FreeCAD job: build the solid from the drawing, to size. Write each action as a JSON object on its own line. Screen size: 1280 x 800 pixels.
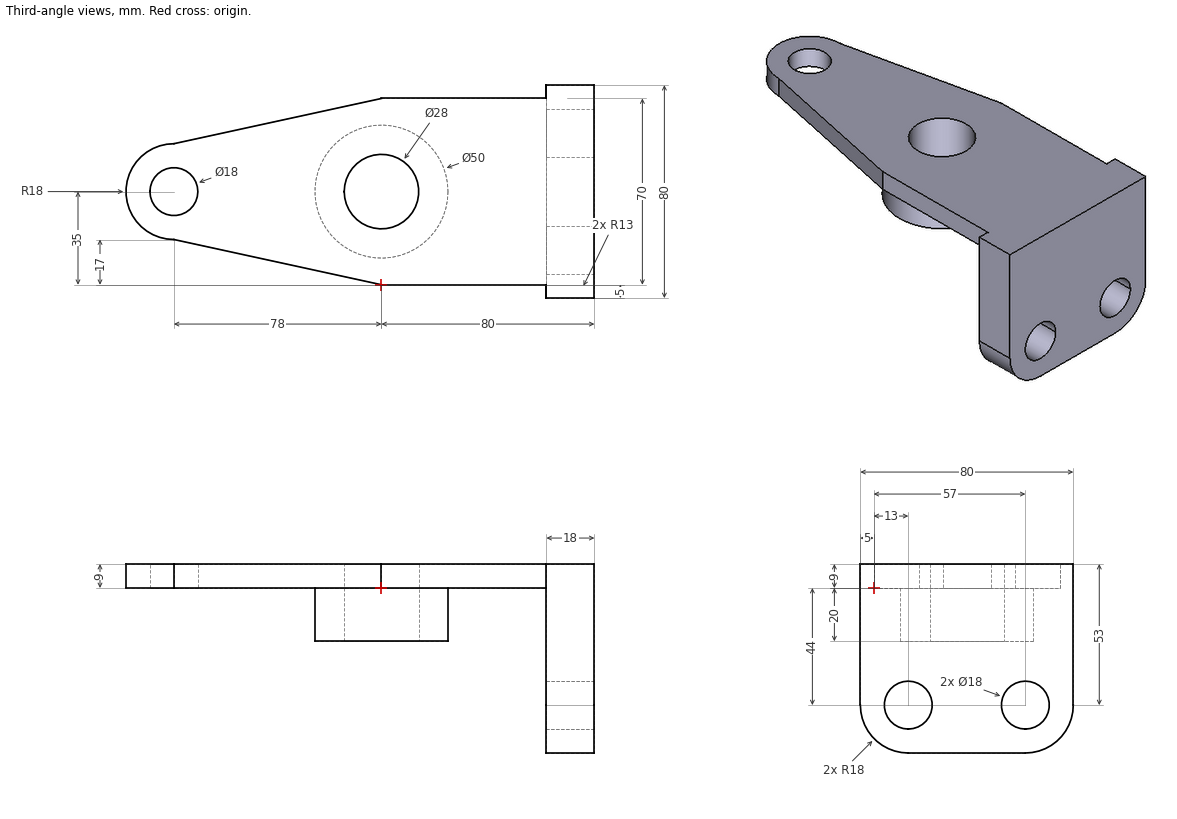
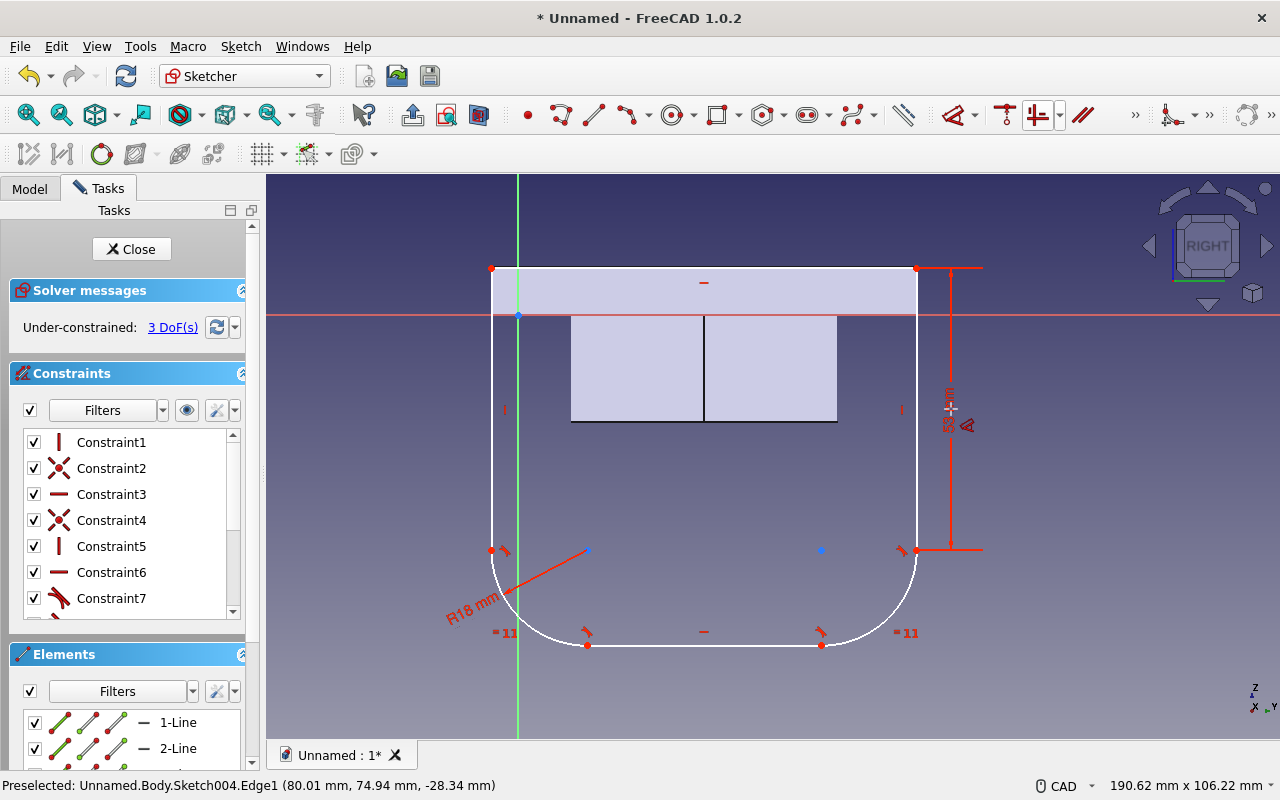
{"action": "left_click", "coordinate": [789, 268]}
{"action": "left_click", "coordinate": [704, 234]}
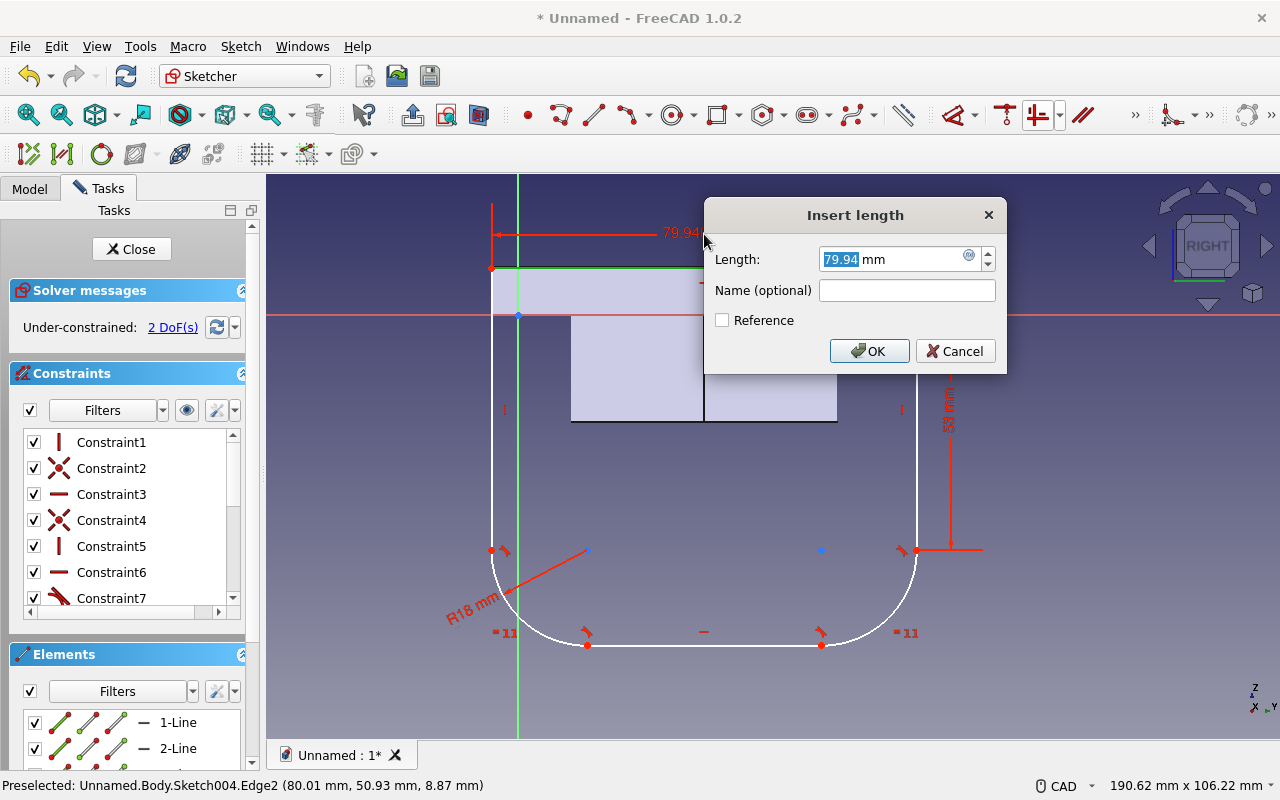
{"action": "type", "text": "80"}
{"action": "key", "text": "Return"}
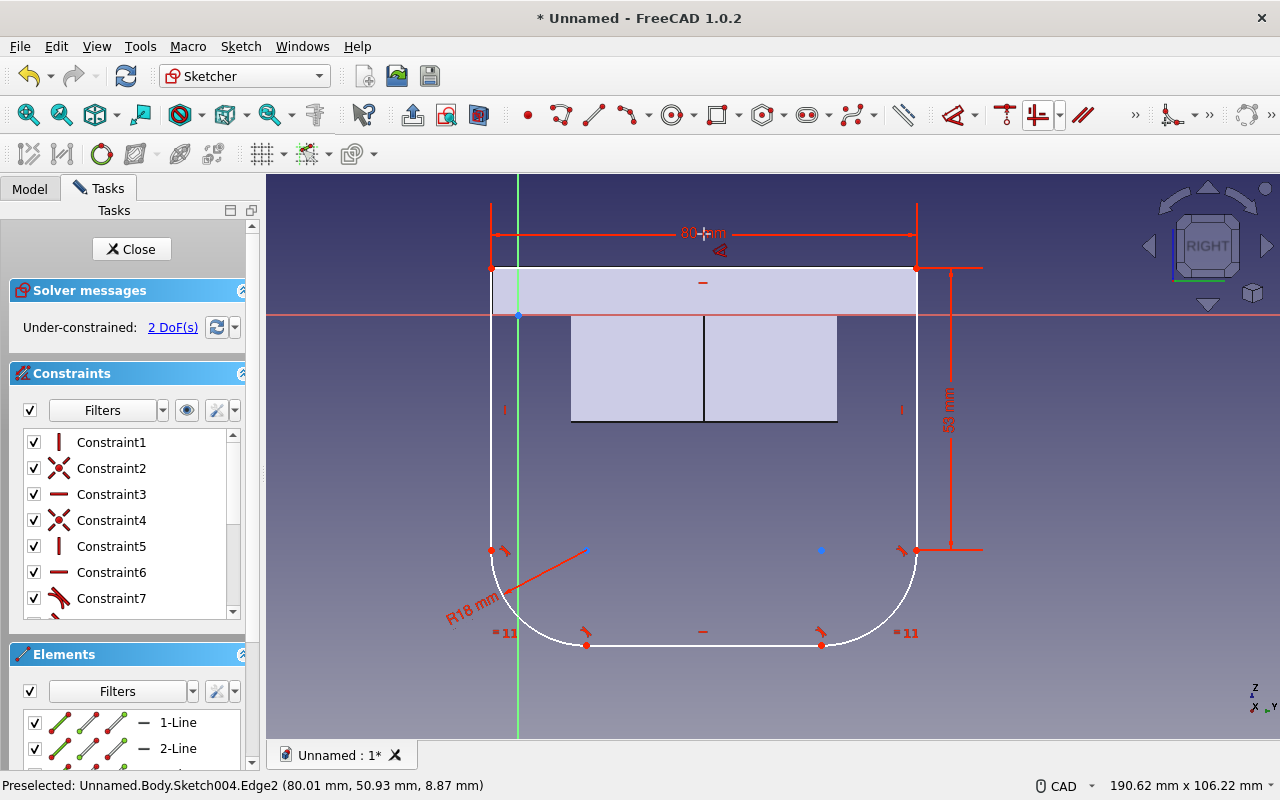
{"action": "left_click", "coordinate": [917, 268]}
{"action": "left_click", "coordinate": [951, 292]}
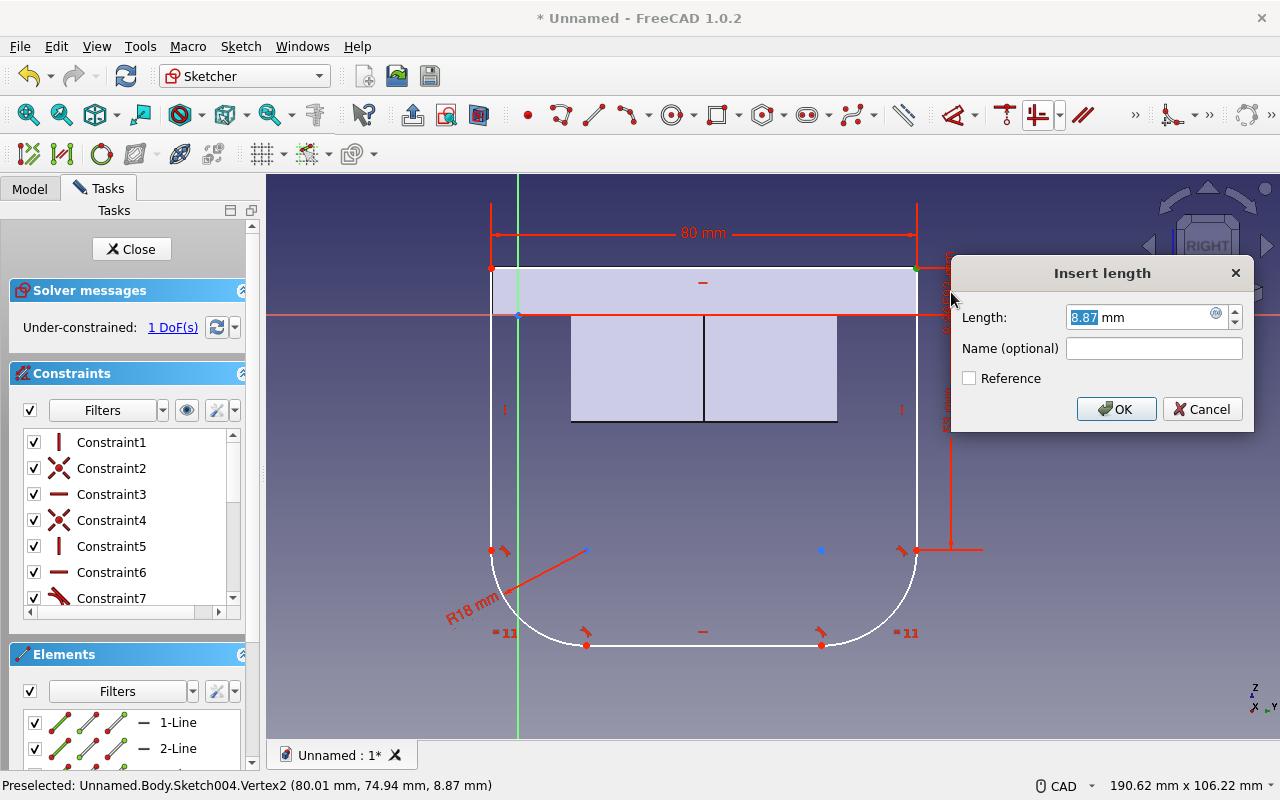
{"action": "type", "text": "9"}
{"action": "key", "text": "Return"}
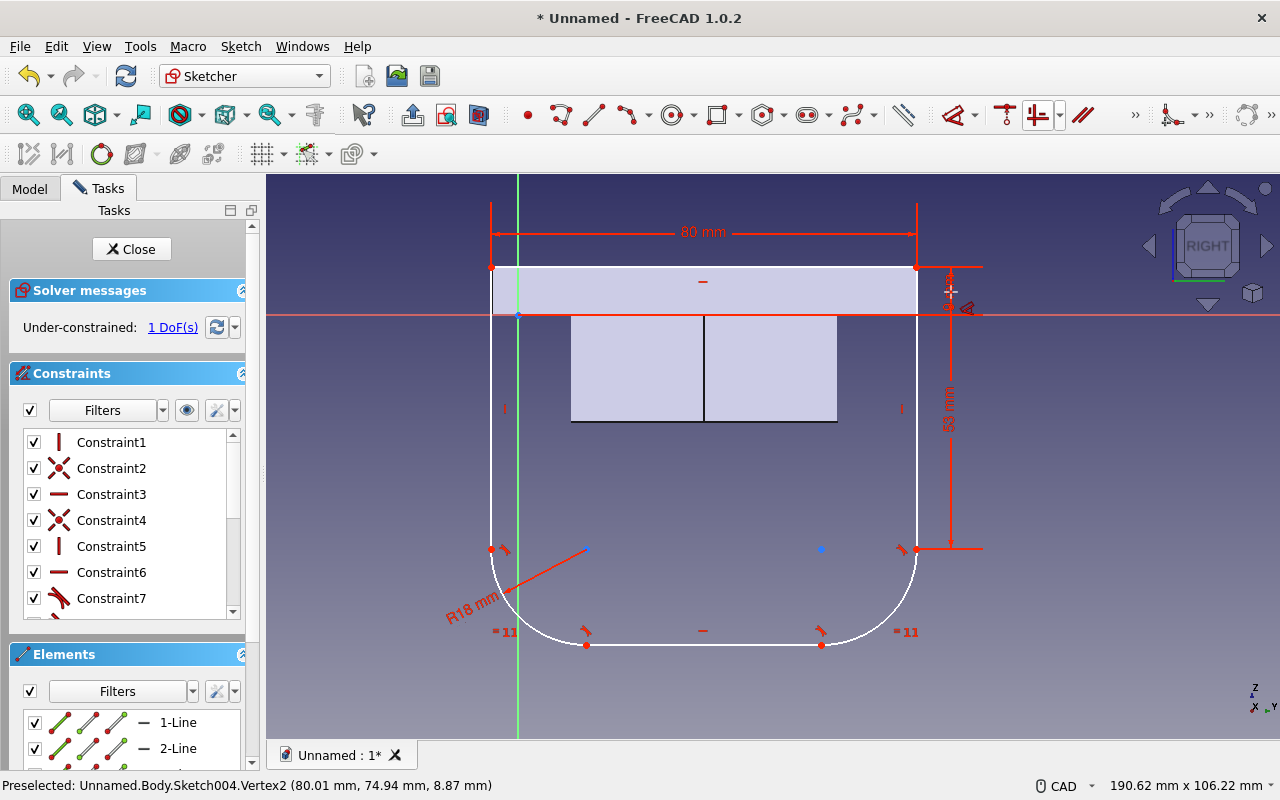
{"action": "scroll", "coordinate": [491, 267], "scroll_direction": "up", "scroll_amount": 3}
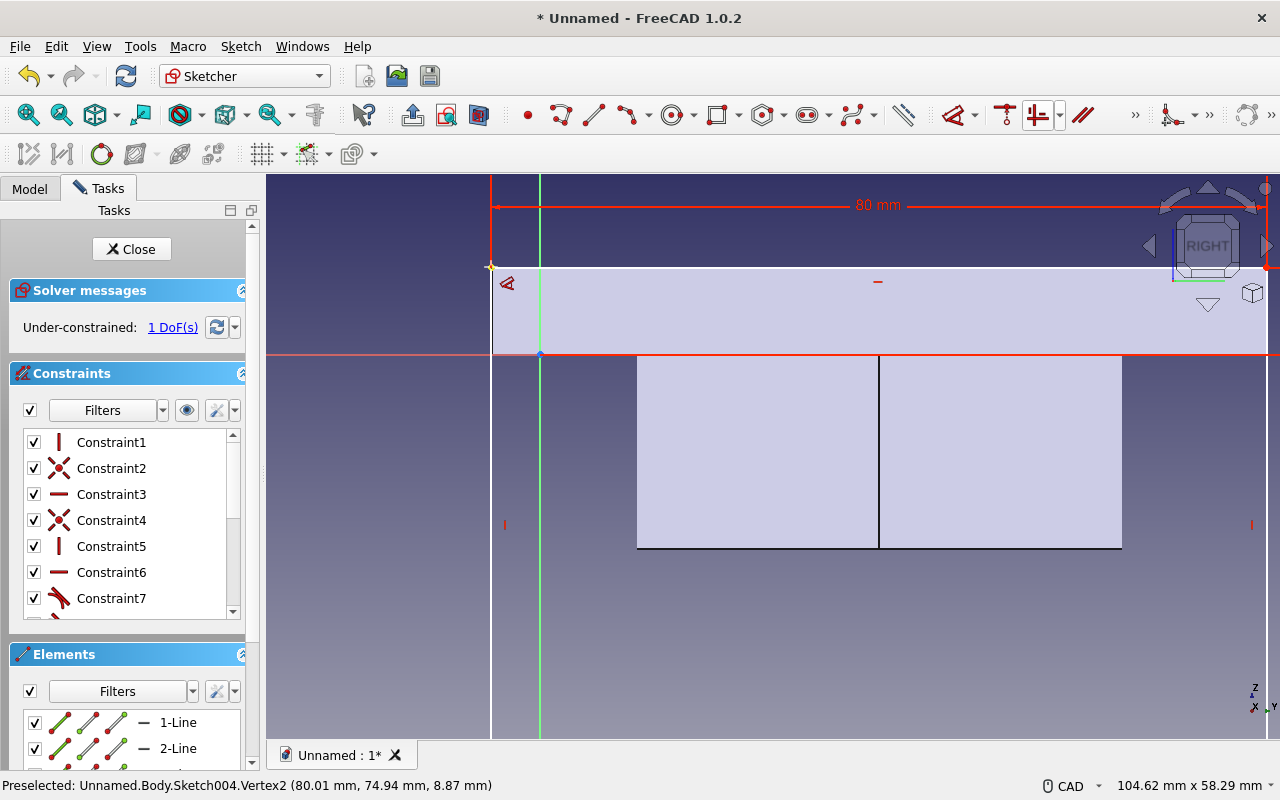
{"action": "left_click", "coordinate": [491, 268]}
{"action": "left_click", "coordinate": [516, 234]}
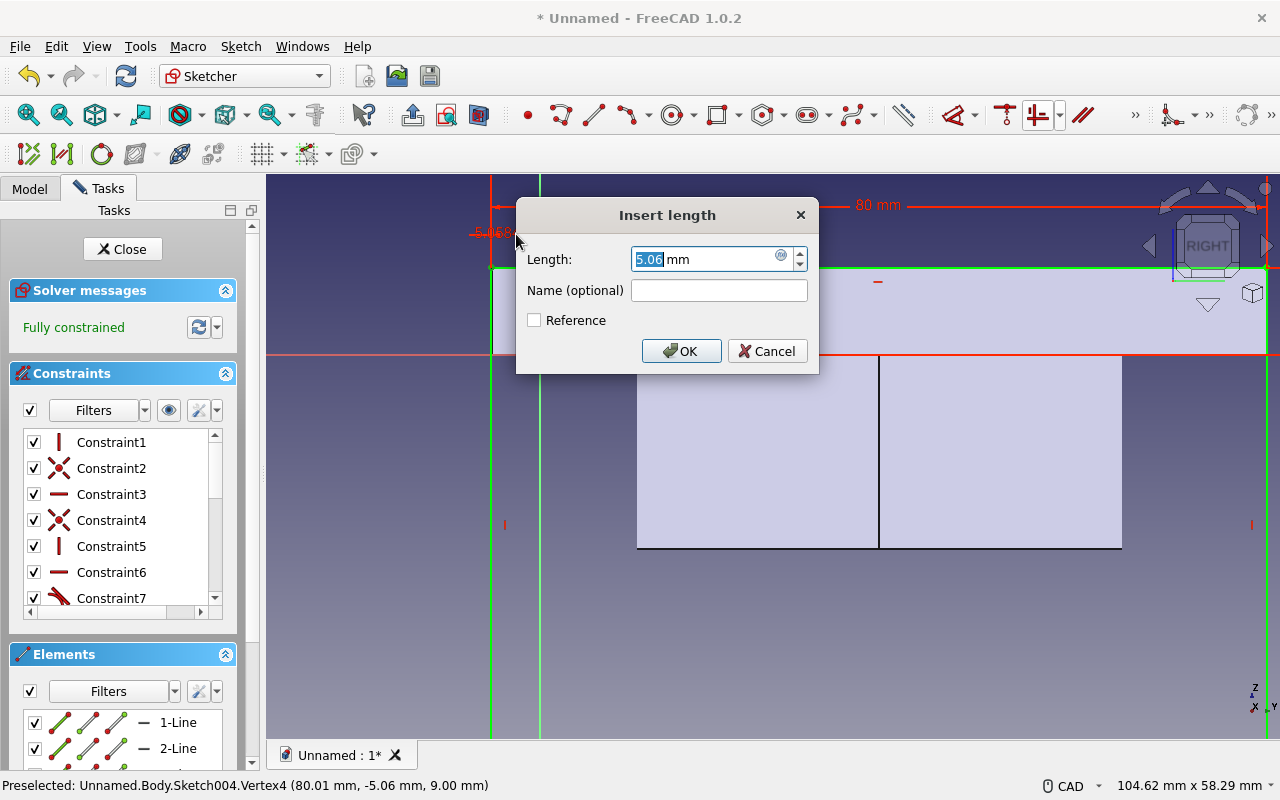
{"action": "type", "text": "5"}
{"action": "key", "text": "Return"}
{"action": "key", "text": "Escape"}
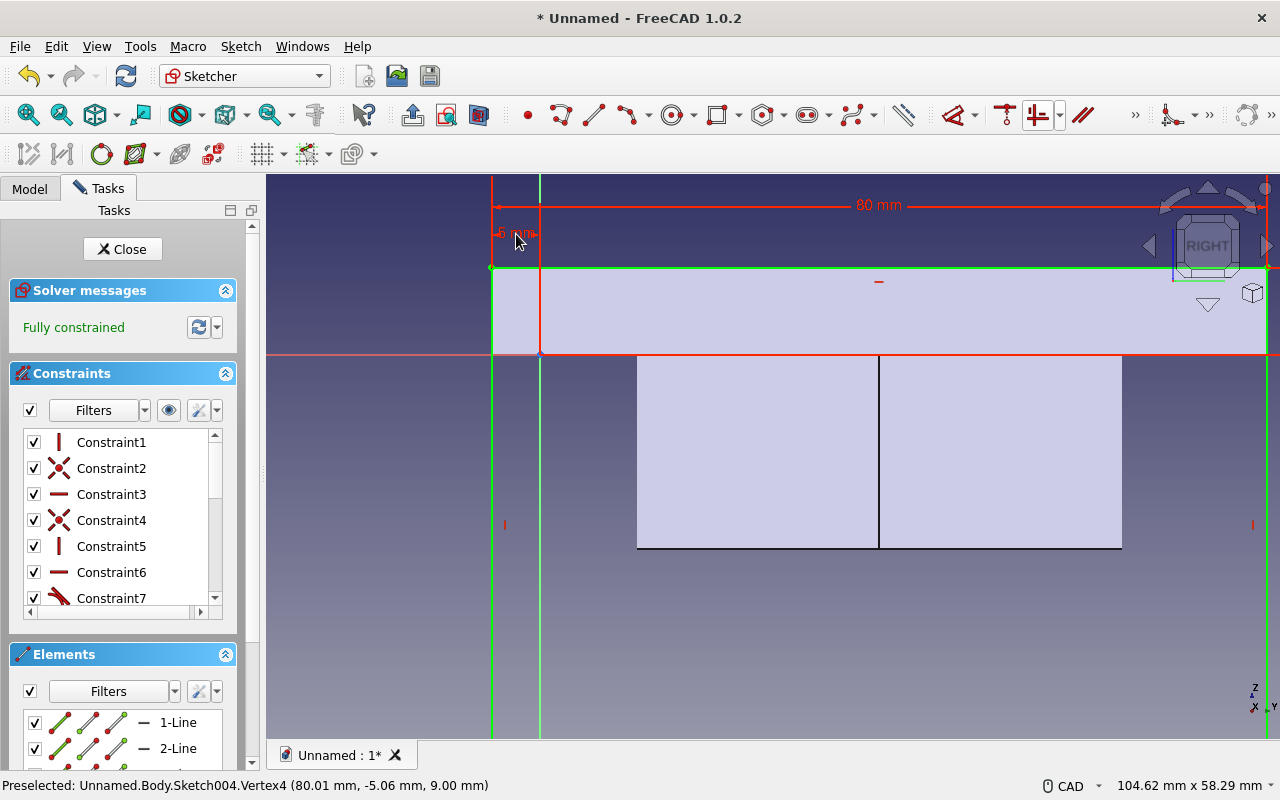
{"action": "left_click", "coordinate": [123, 249]}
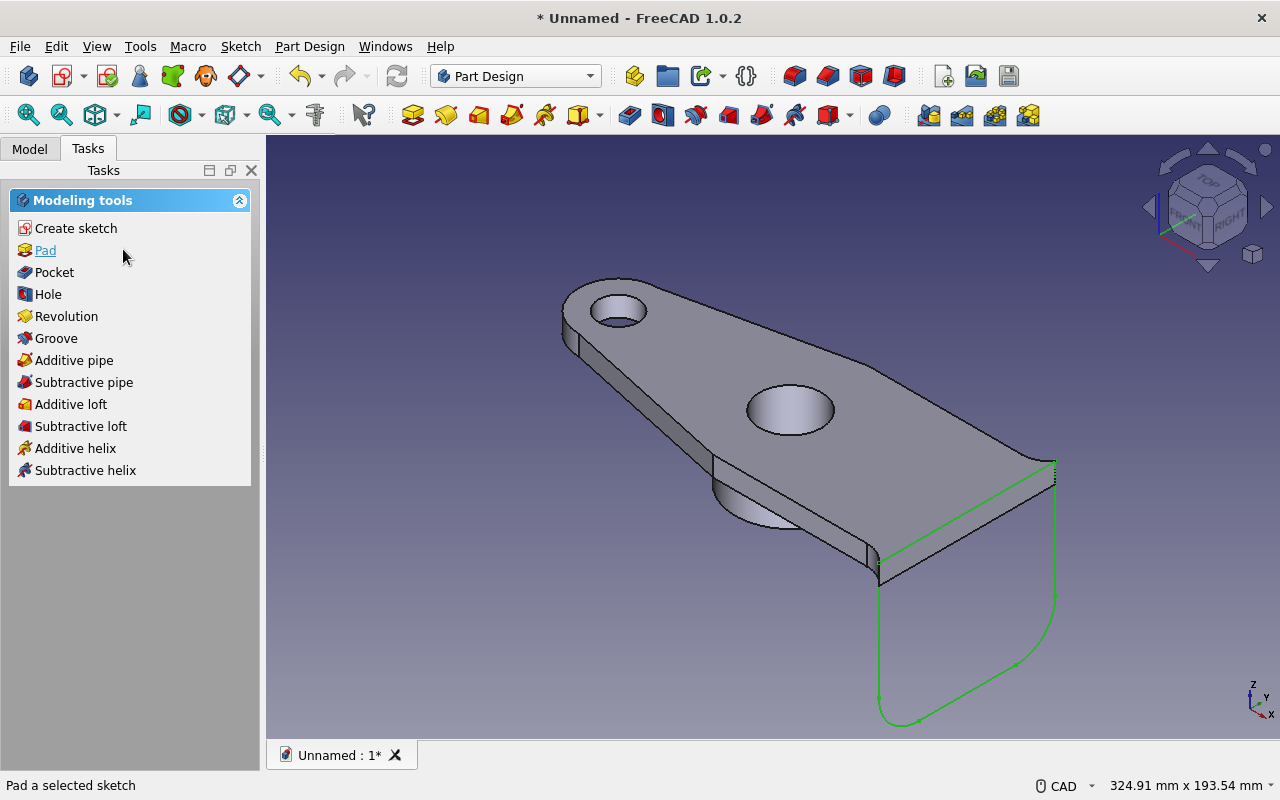
{"action": "left_click", "coordinate": [413, 116]}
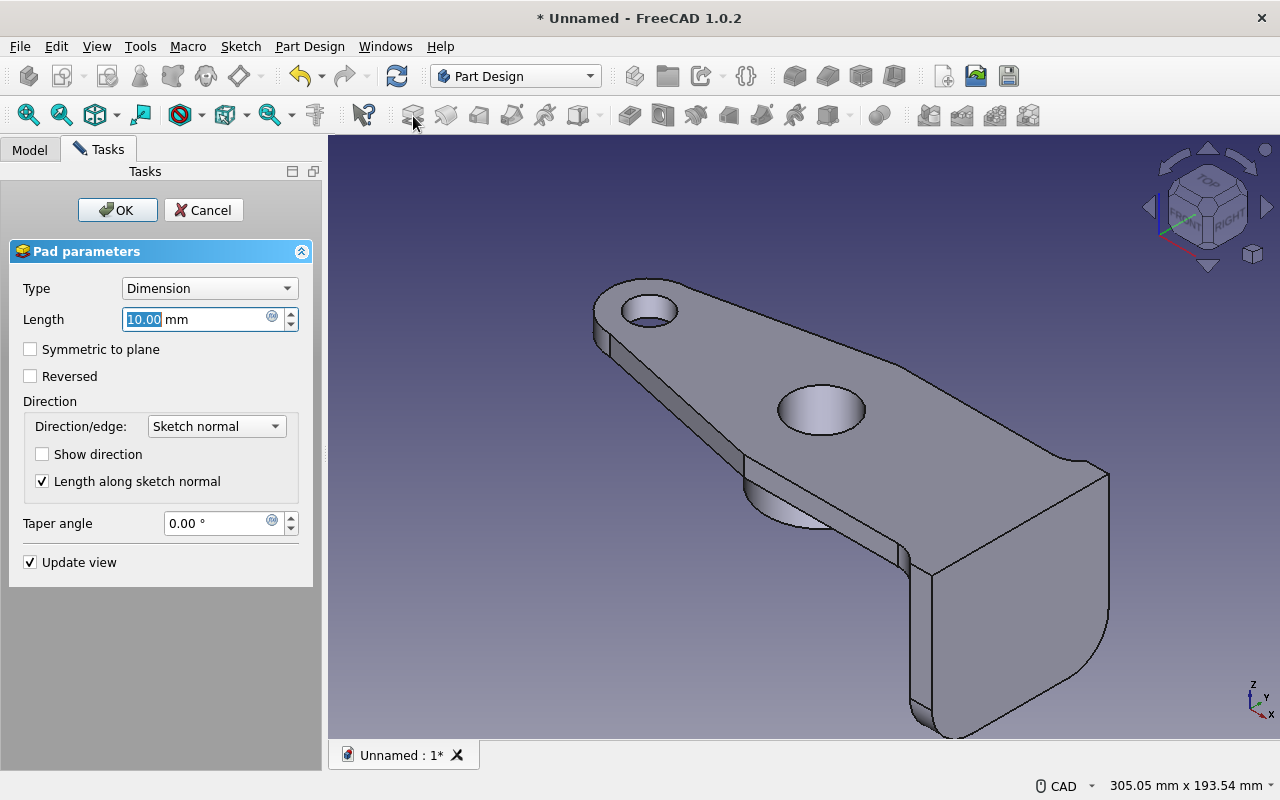
{"action": "type", "text": "18"}
{"action": "key", "text": "Tab"}